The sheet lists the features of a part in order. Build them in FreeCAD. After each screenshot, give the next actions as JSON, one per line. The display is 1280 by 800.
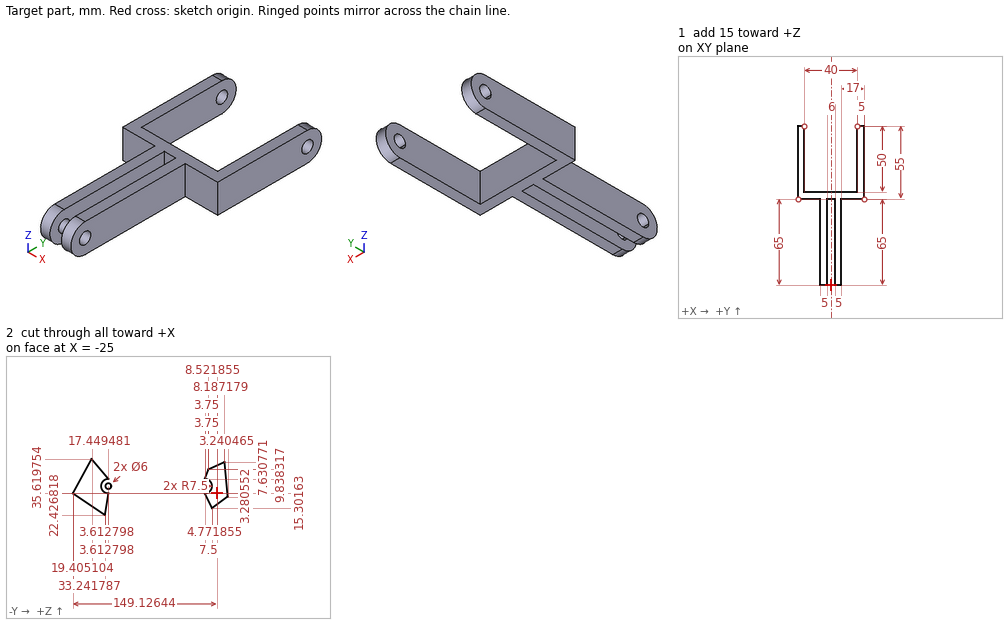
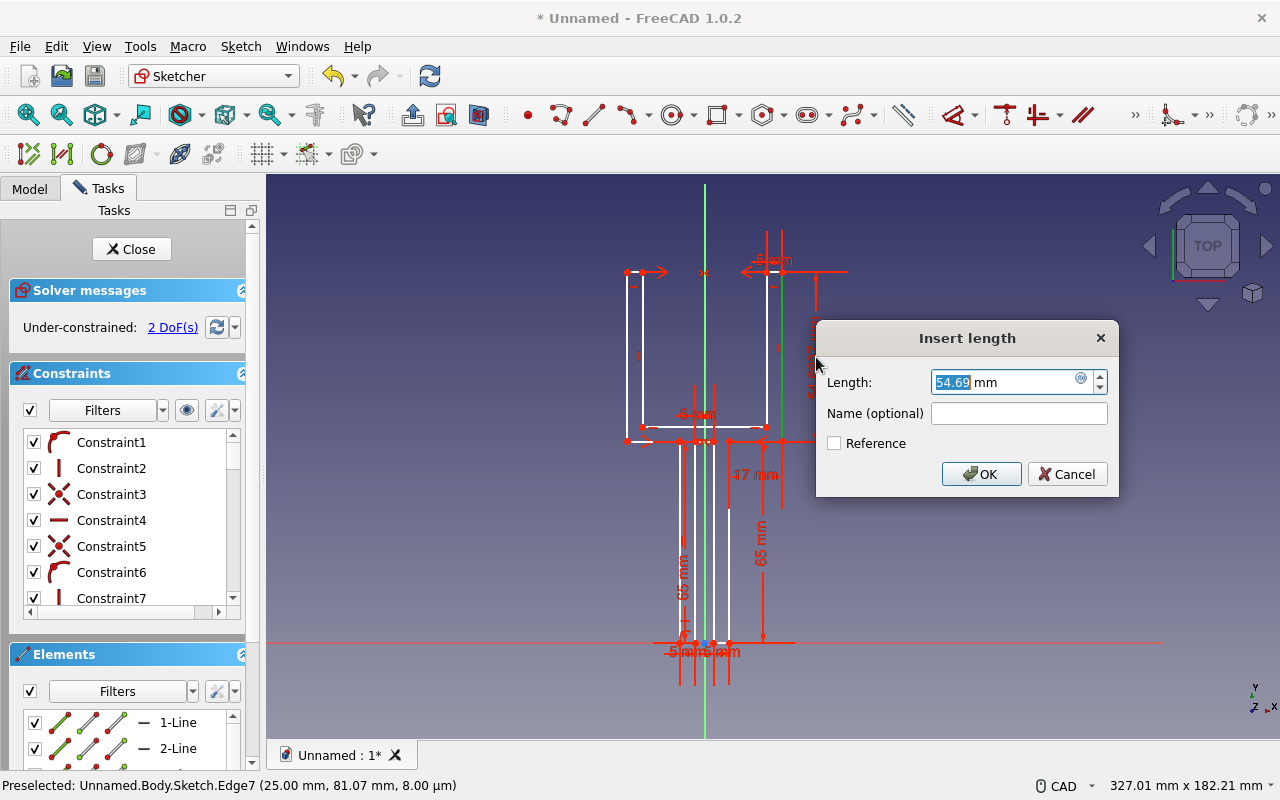
{"action": "type", "text": "55"}
{"action": "key", "text": "Return"}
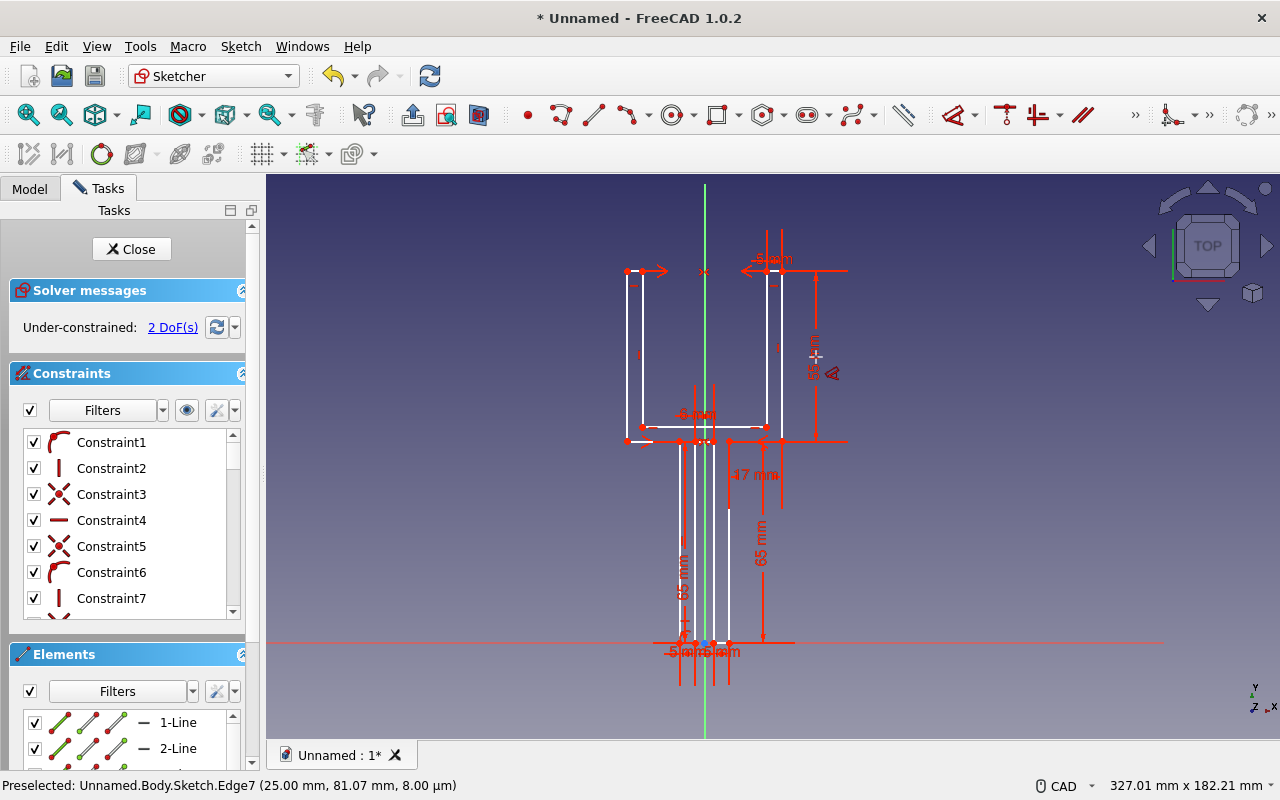
{"action": "left_click", "coordinate": [767, 318]}
{"action": "left_click", "coordinate": [801, 313]}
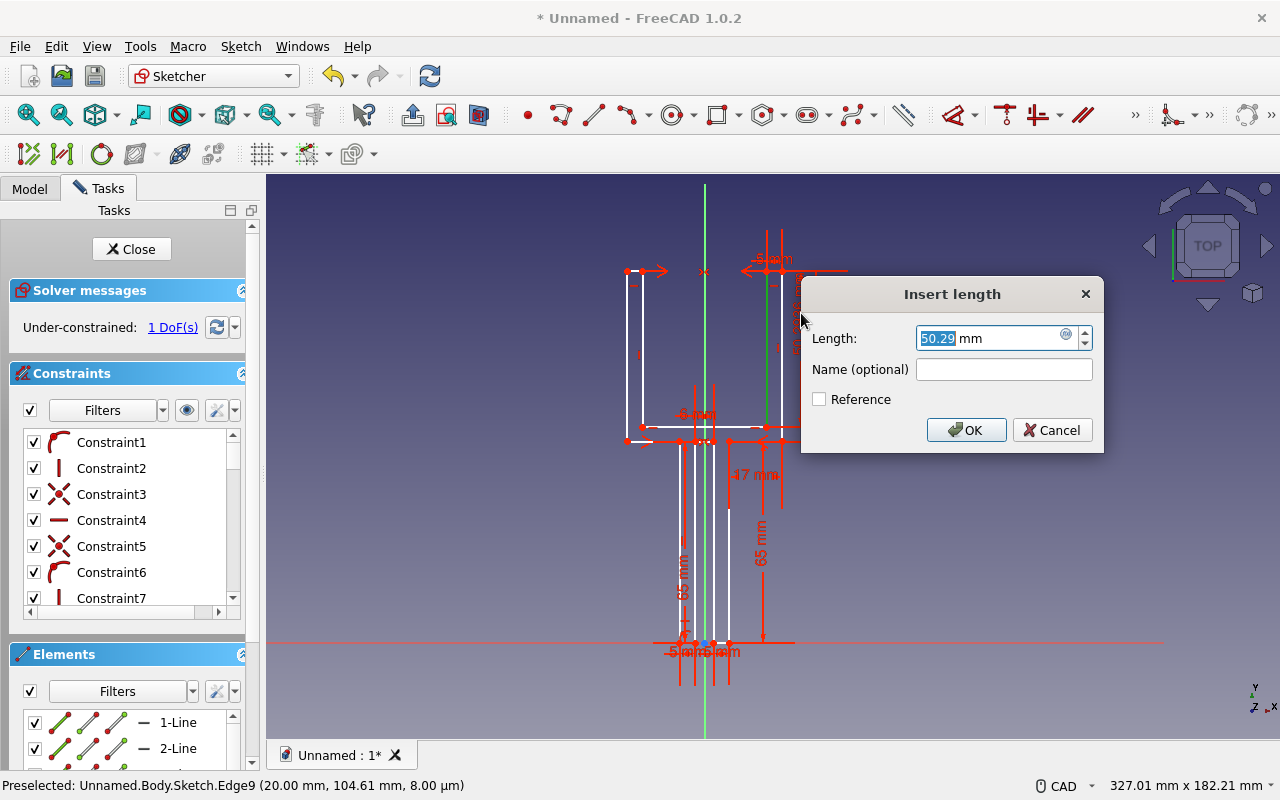
{"action": "type", "text": "50"}
{"action": "key", "text": "Return"}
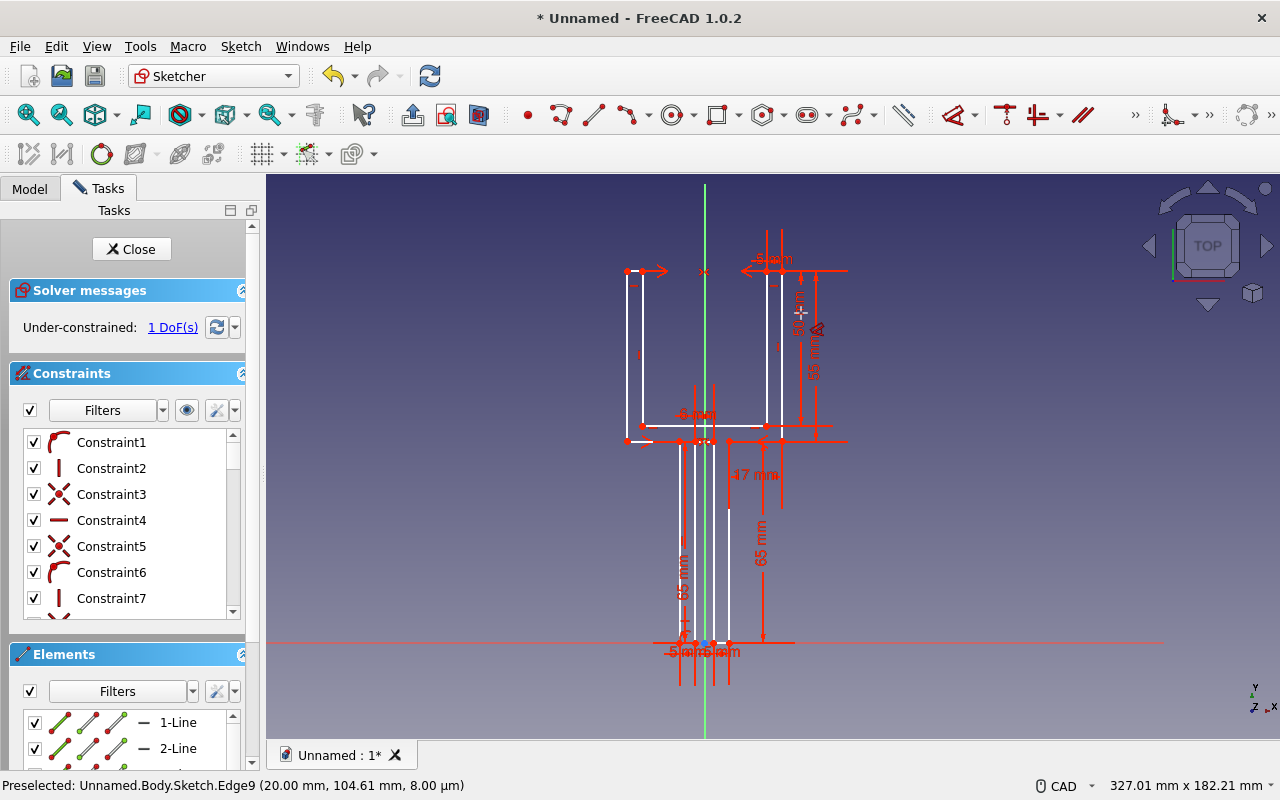
{"action": "left_click", "coordinate": [729, 426]}
{"action": "left_click", "coordinate": [676, 392]}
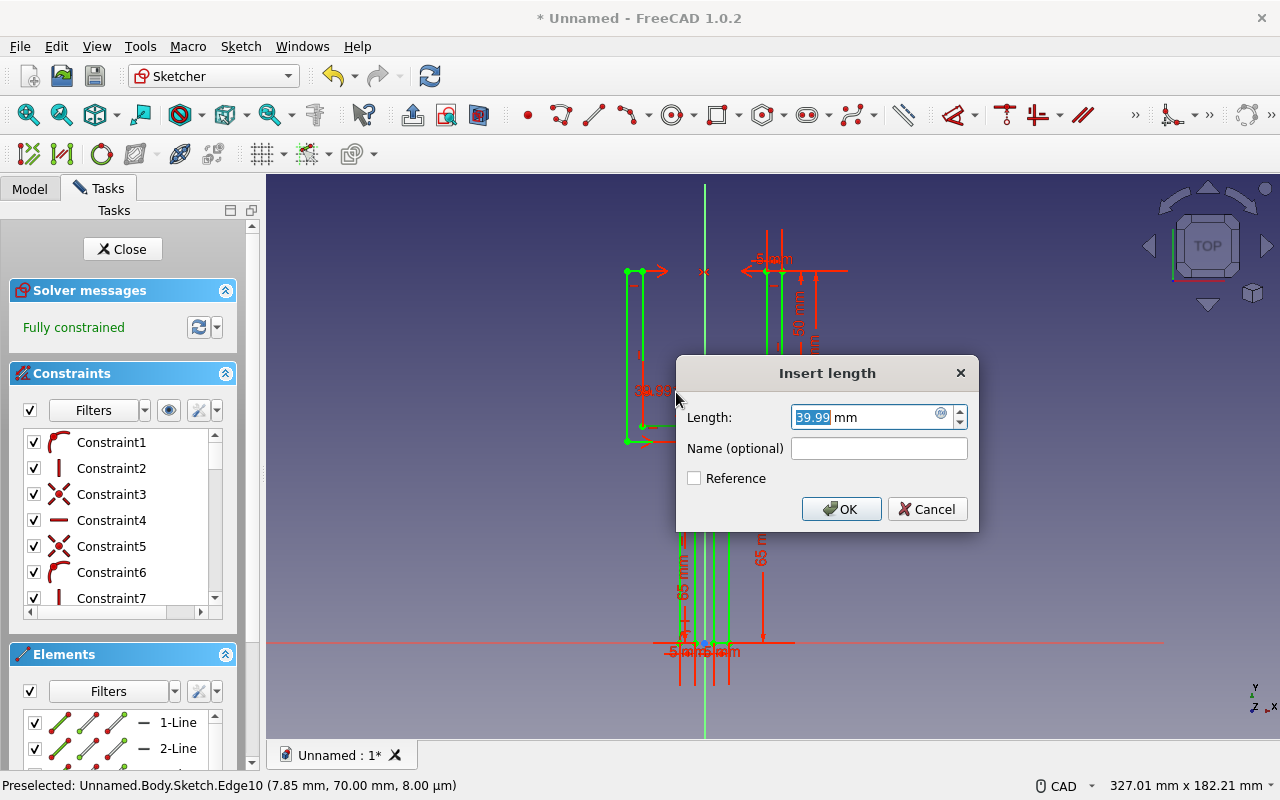
{"action": "type", "text": "40"}
{"action": "key", "text": "Return"}
{"action": "key", "text": "Escape"}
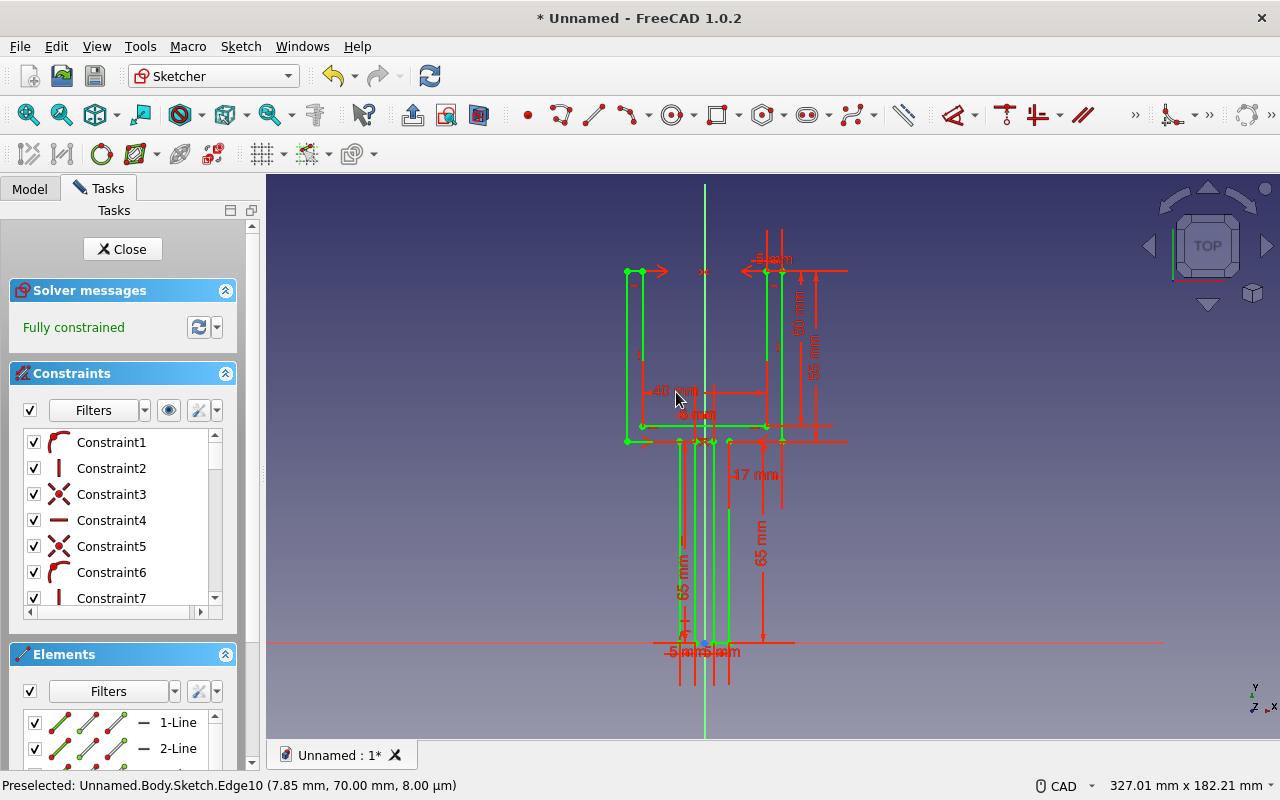
{"action": "left_click", "coordinate": [123, 249]}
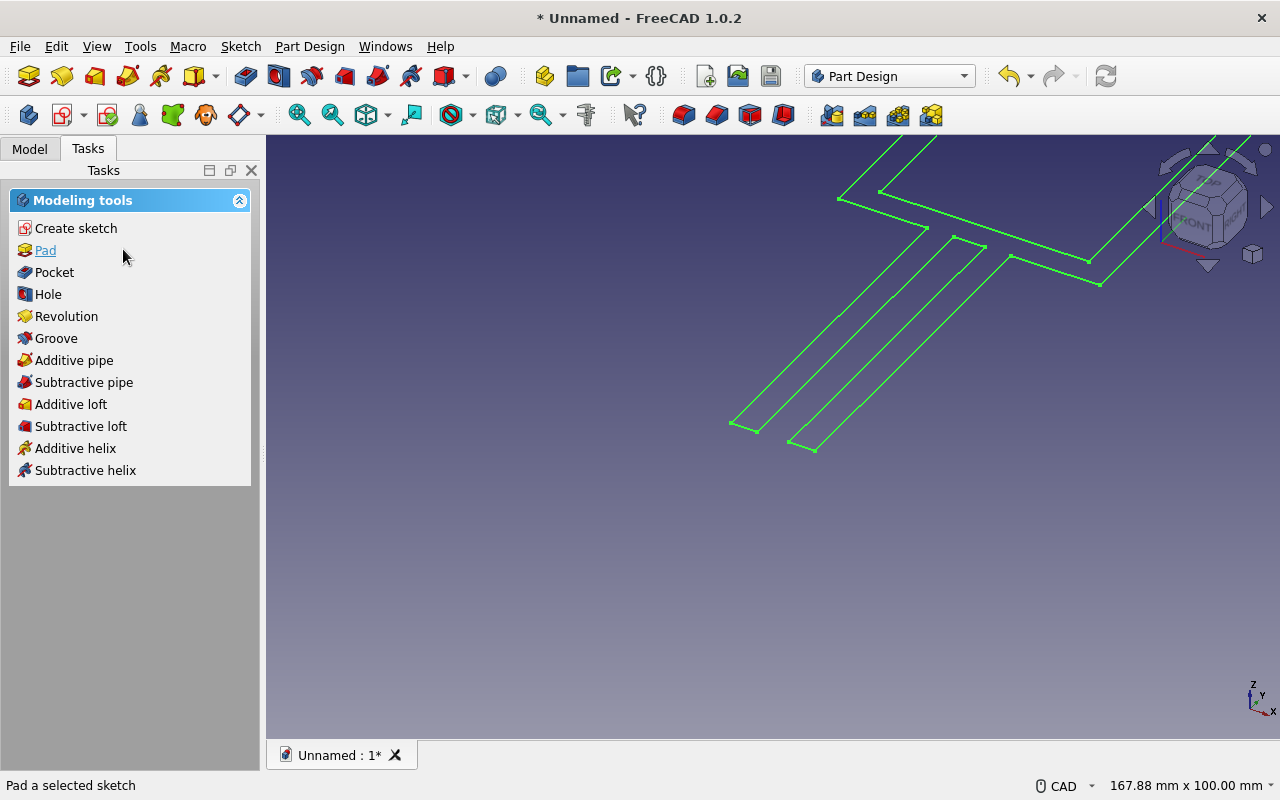
{"action": "left_click", "coordinate": [29, 76]}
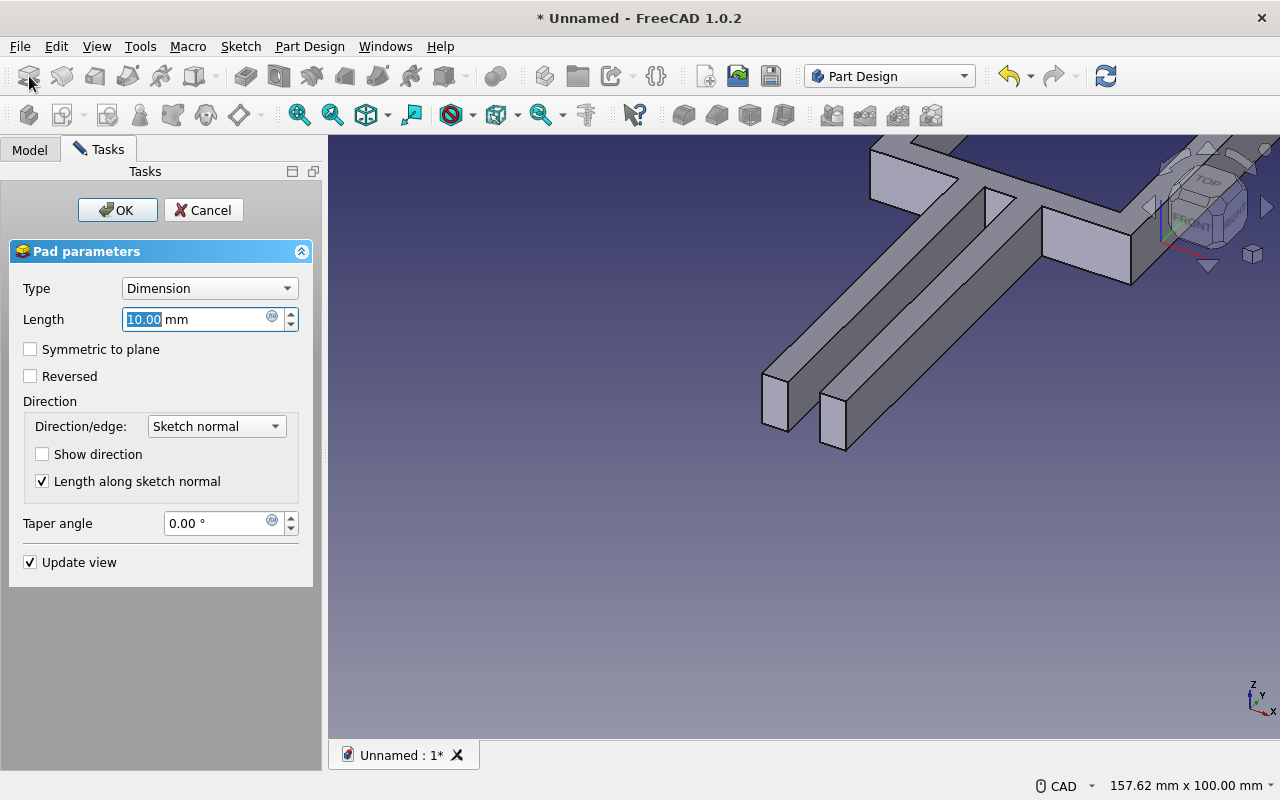
{"action": "type", "text": "15"}
{"action": "key", "text": "Tab"}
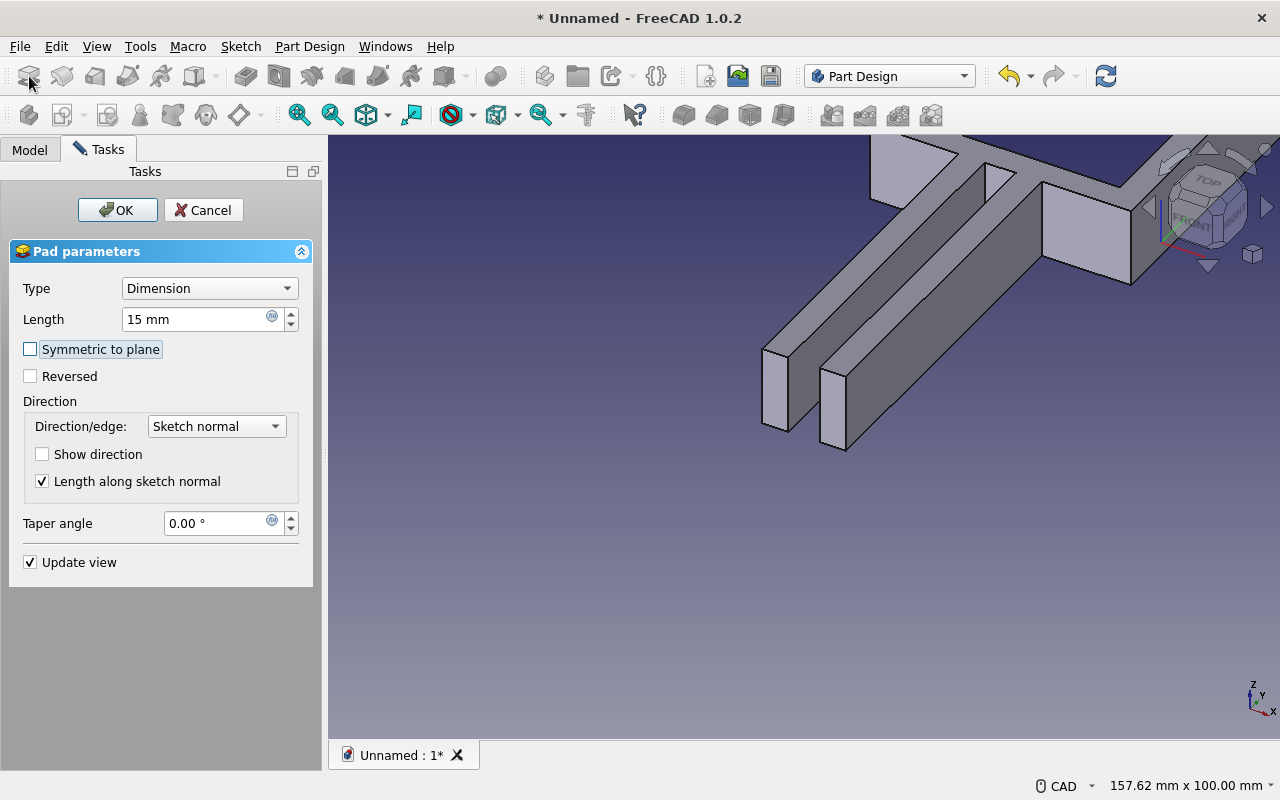
{"action": "left_click", "coordinate": [118, 210]}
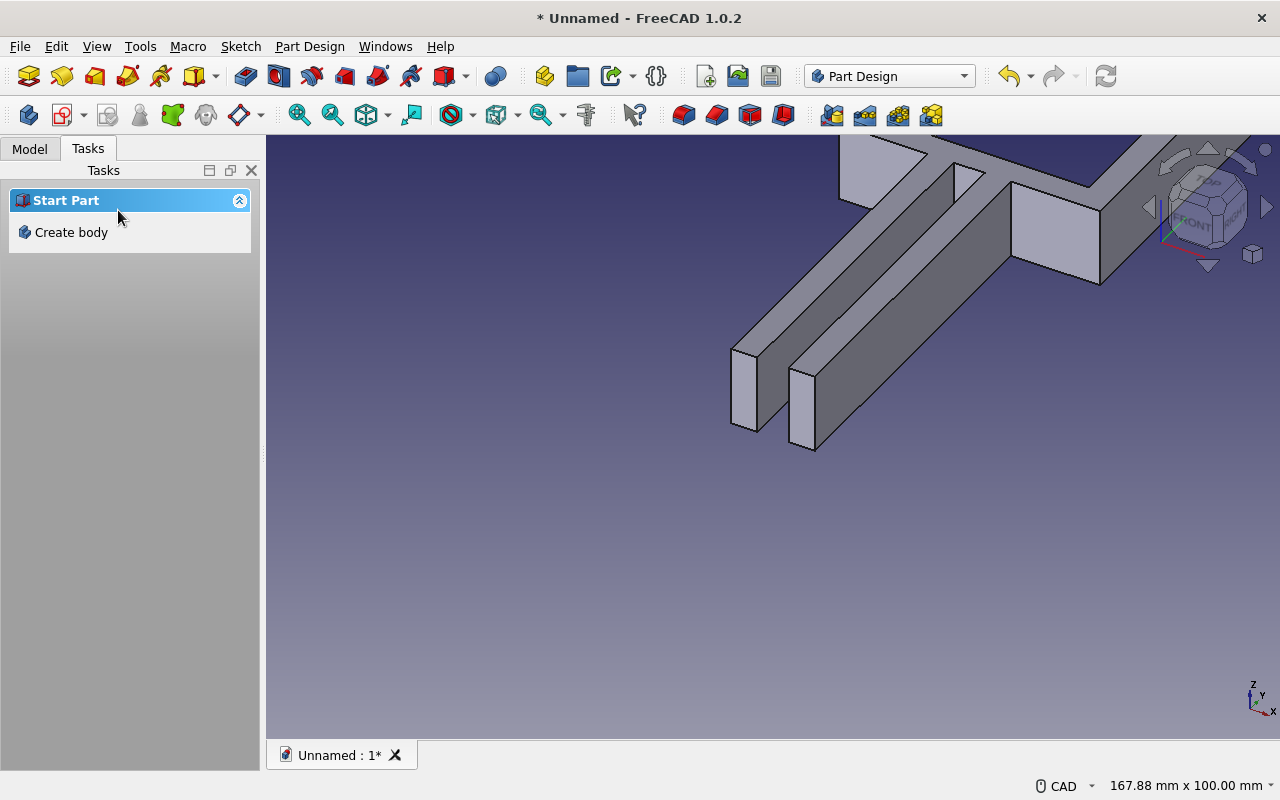
{"action": "left_click", "coordinate": [300, 116]}